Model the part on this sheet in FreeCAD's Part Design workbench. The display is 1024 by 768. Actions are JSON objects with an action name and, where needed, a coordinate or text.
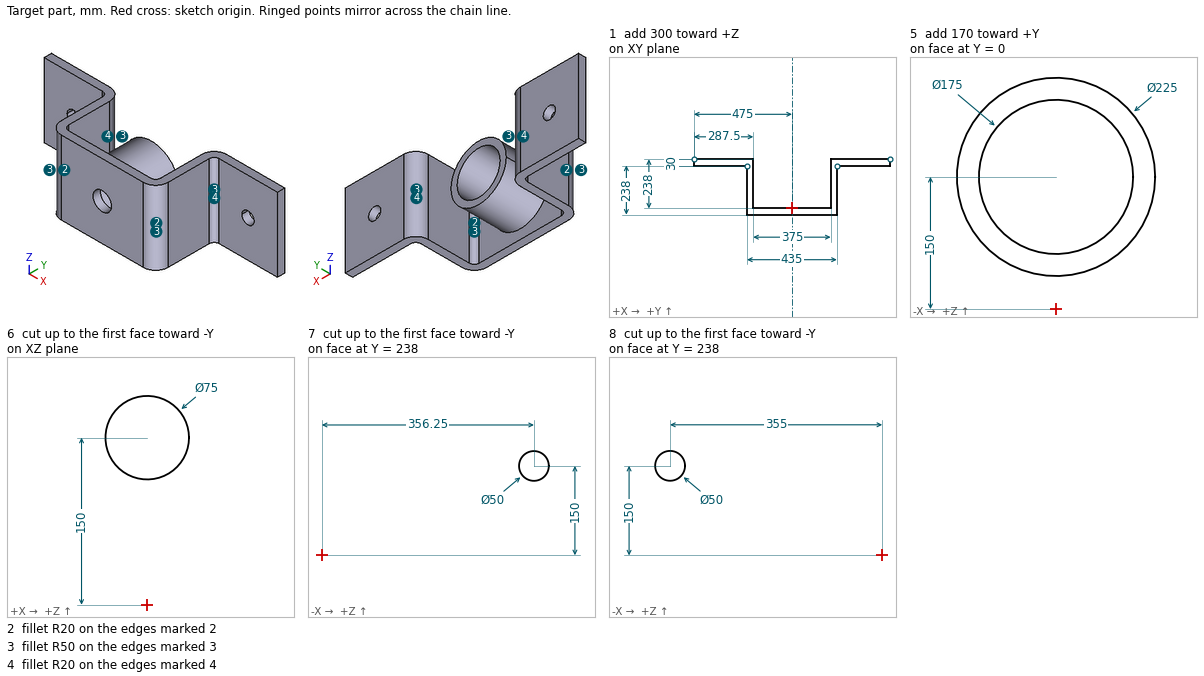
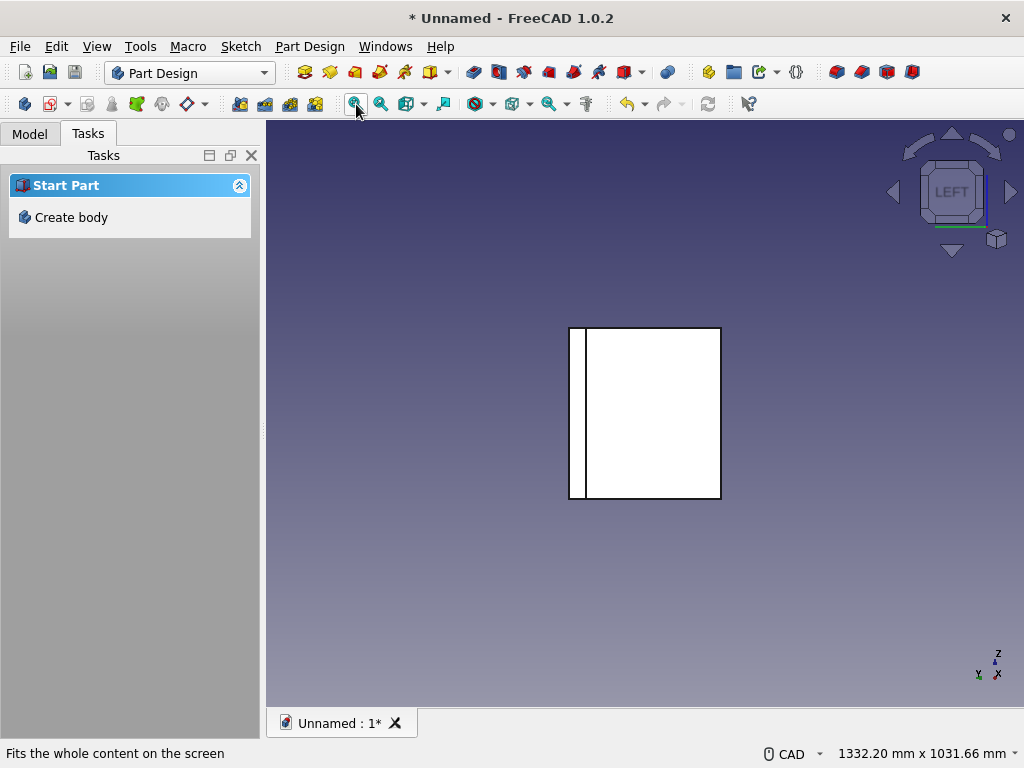
{"action": "key", "text": "v 3"}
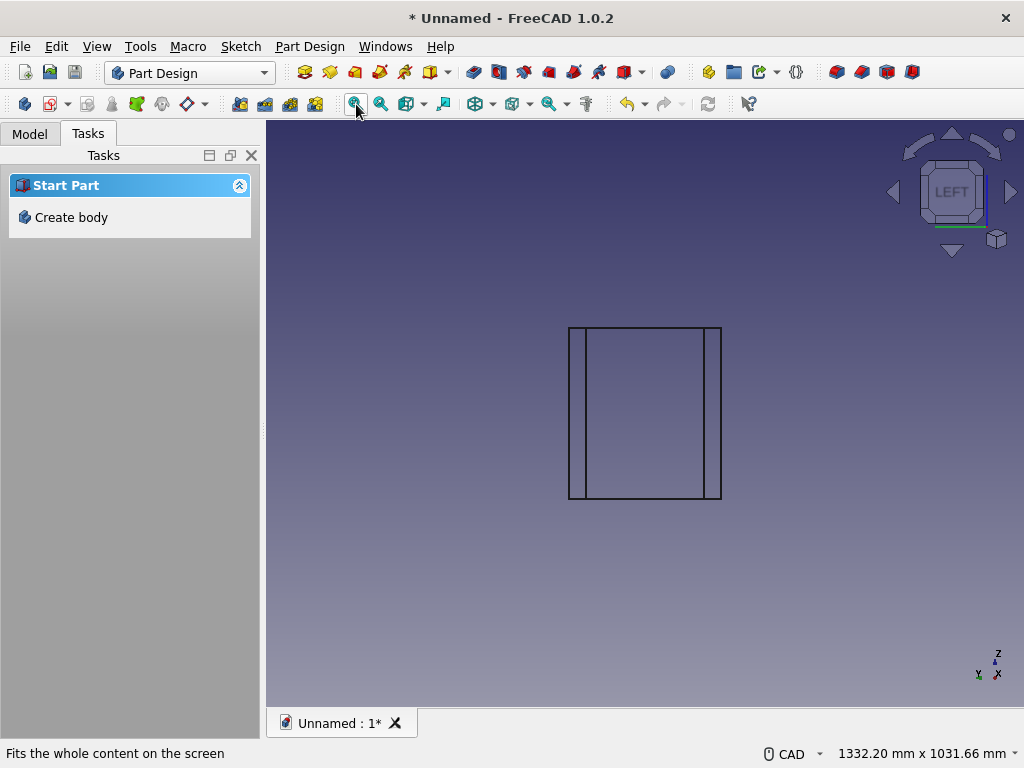
{"action": "key", "text": "0"}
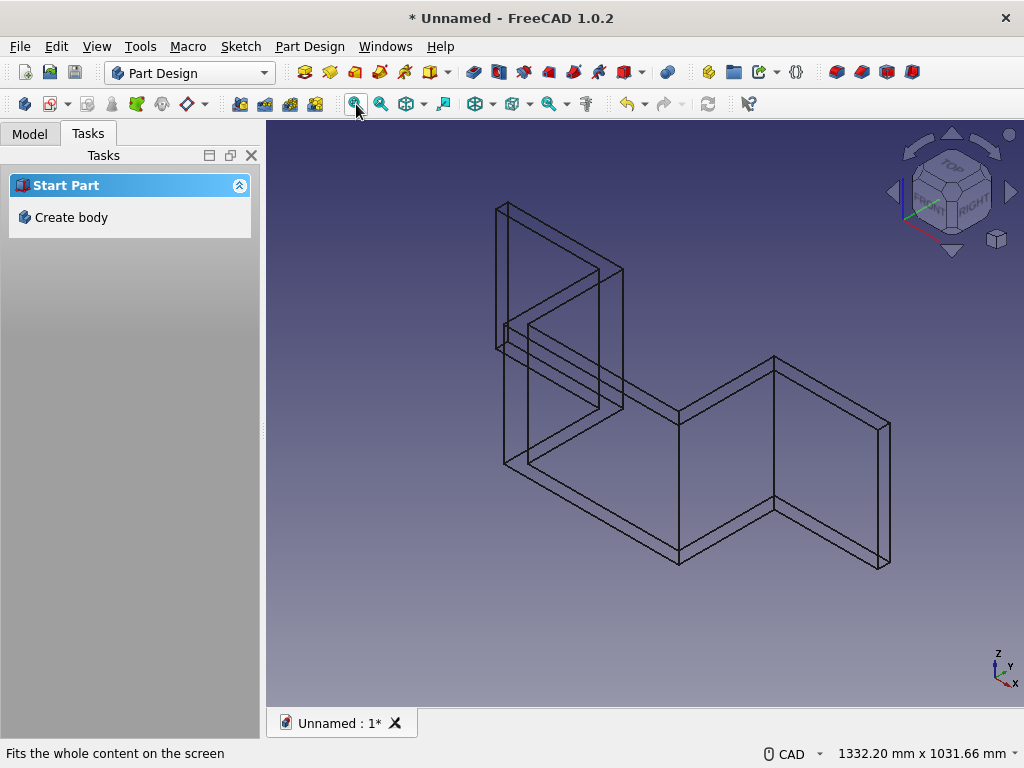
{"action": "left_click", "coordinate": [528, 393]}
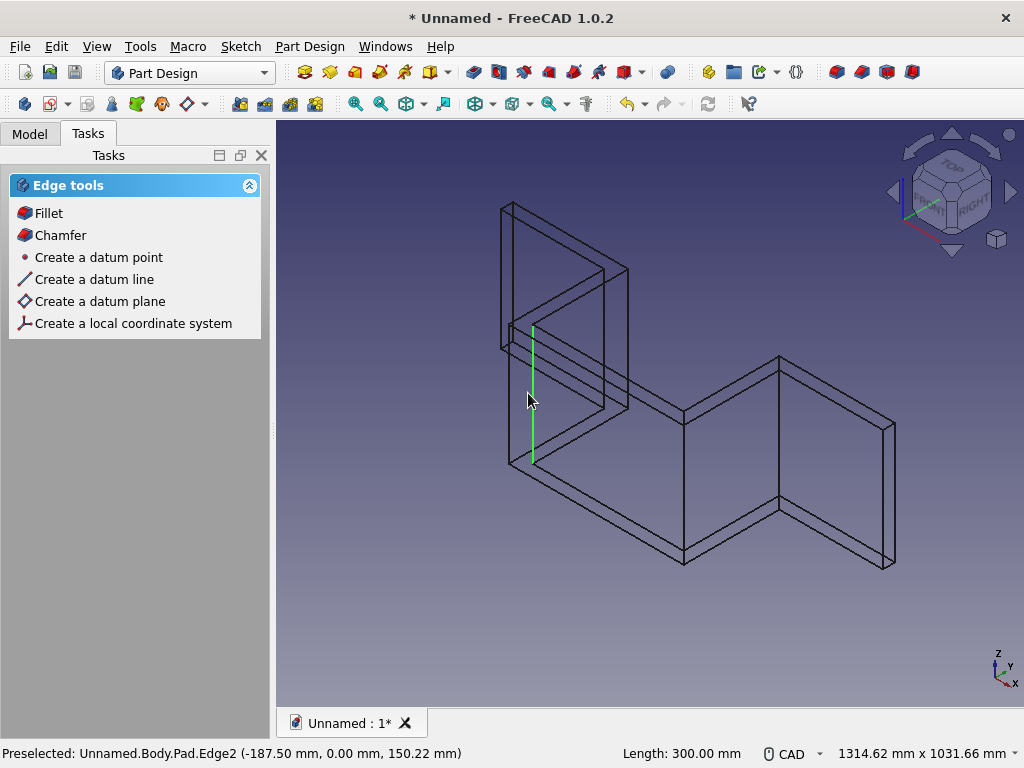
{"action": "scroll", "coordinate": [684, 480], "scroll_direction": "up", "scroll_amount": 6}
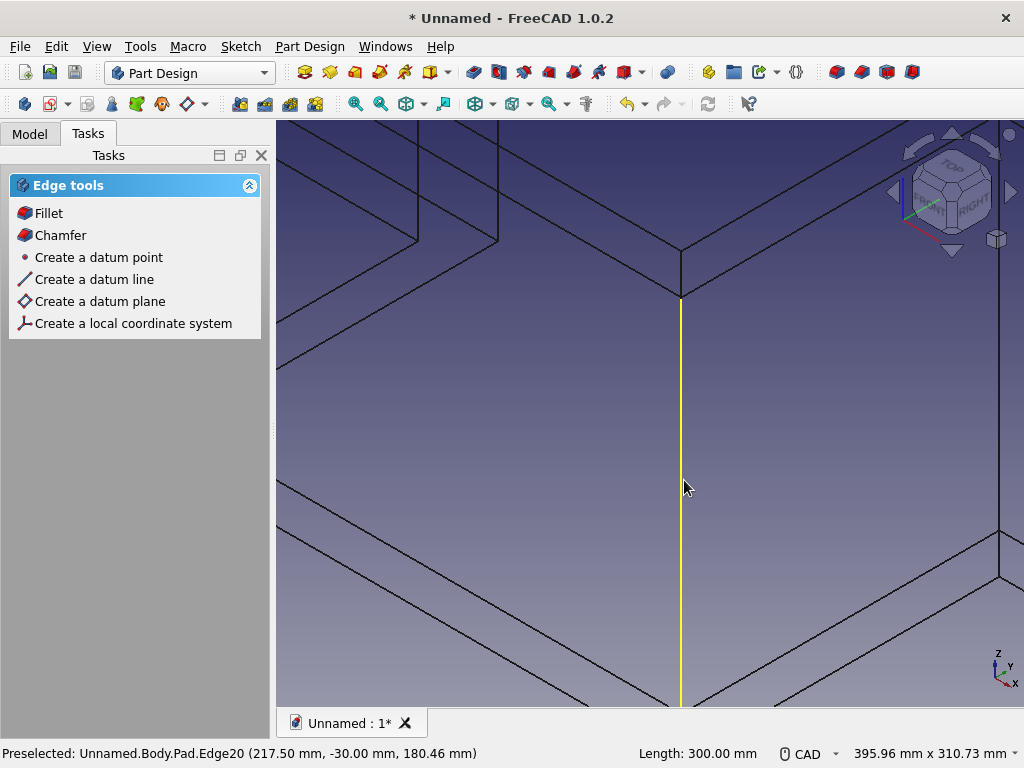
{"action": "left_click", "coordinate": [356, 104]}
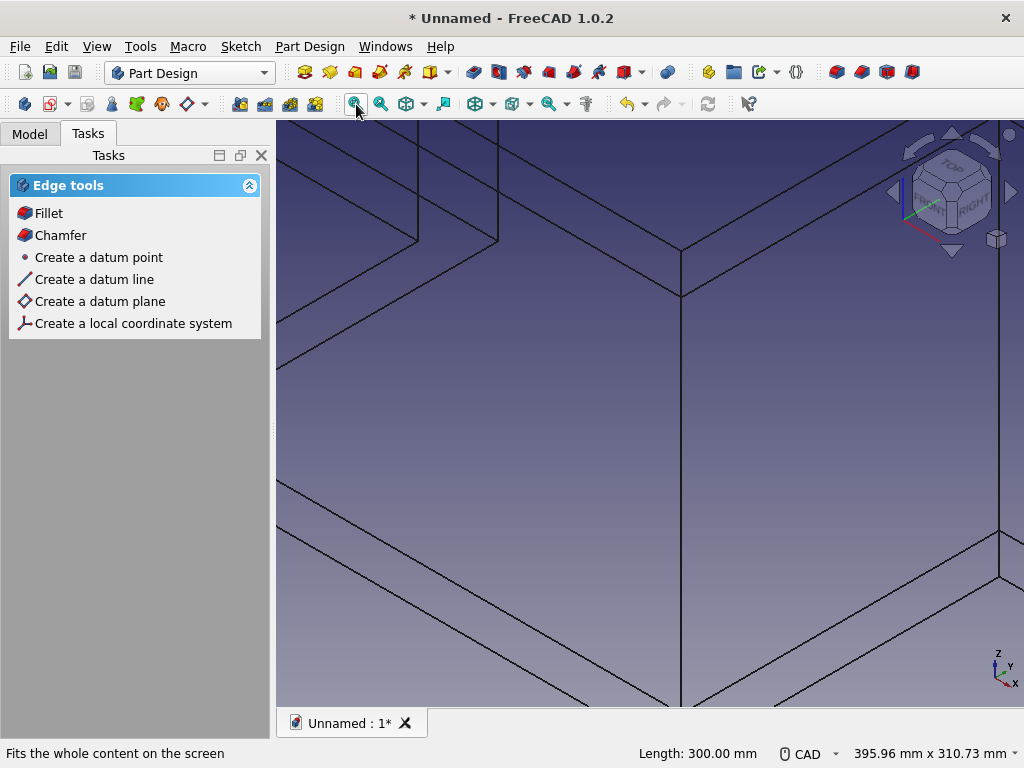
{"action": "key", "text": "2"}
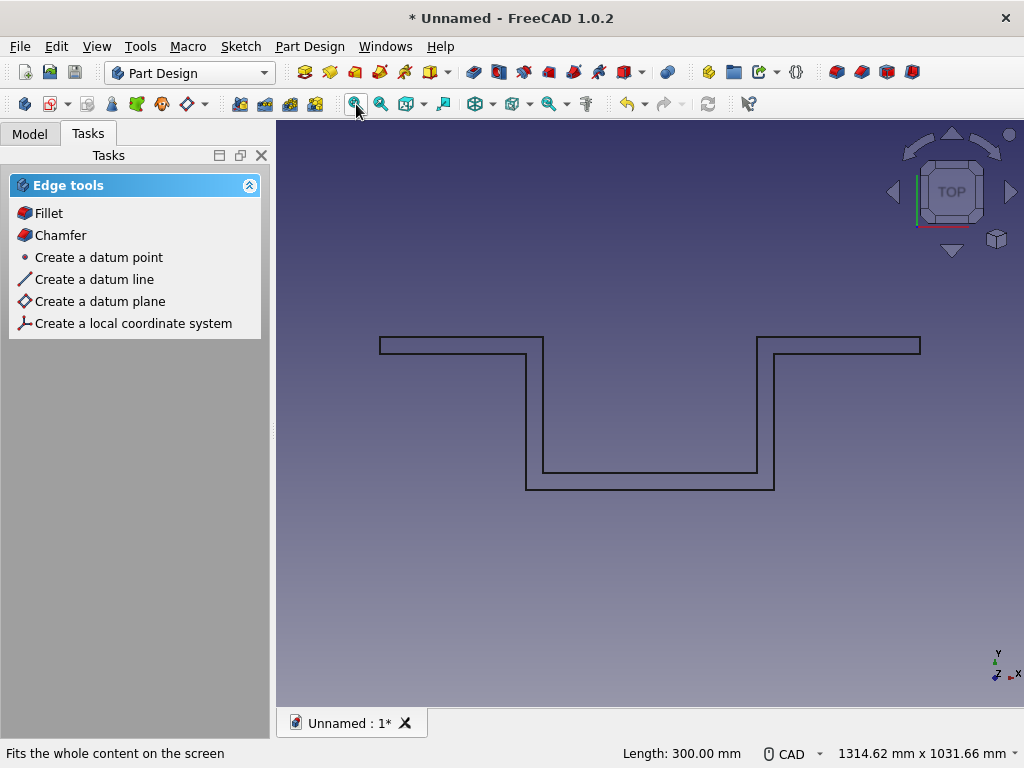
{"action": "scroll", "coordinate": [757, 472], "scroll_direction": "up", "scroll_amount": 6}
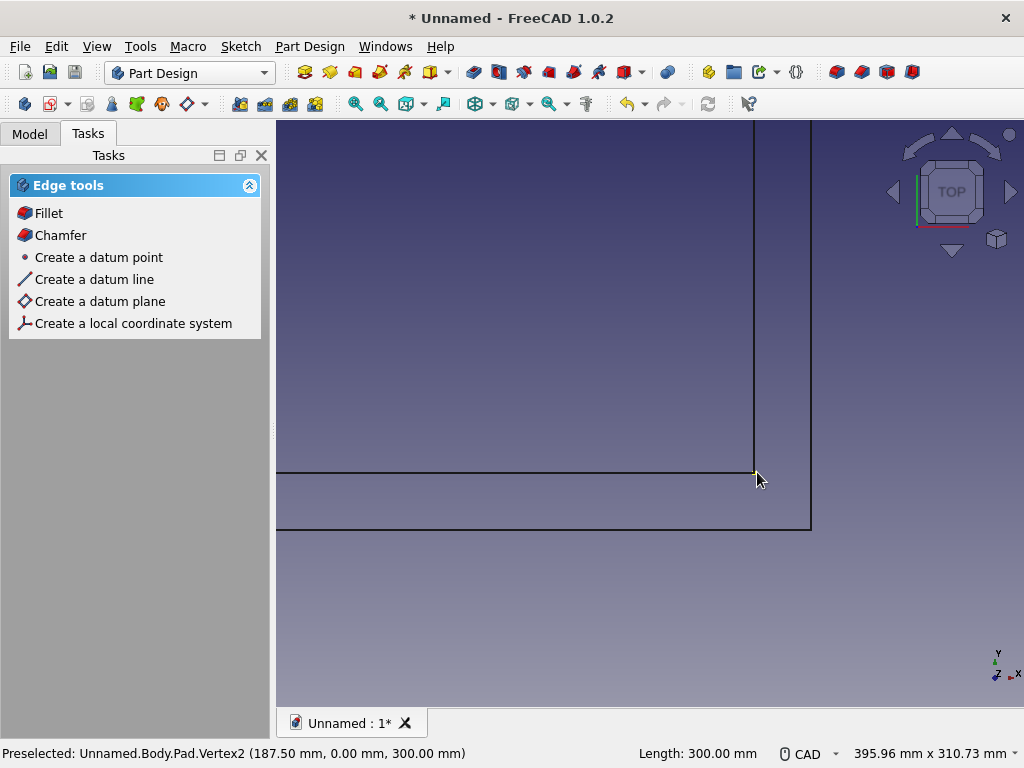
{"action": "left_click", "coordinate": [356, 104]}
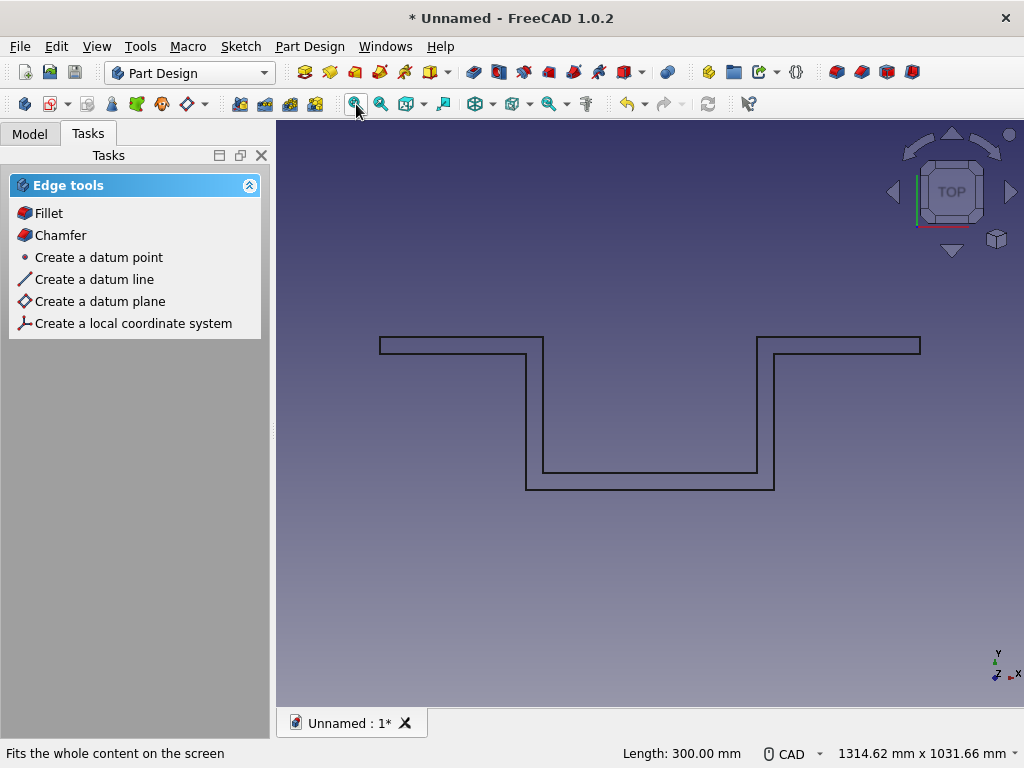
{"action": "key", "text": "1"}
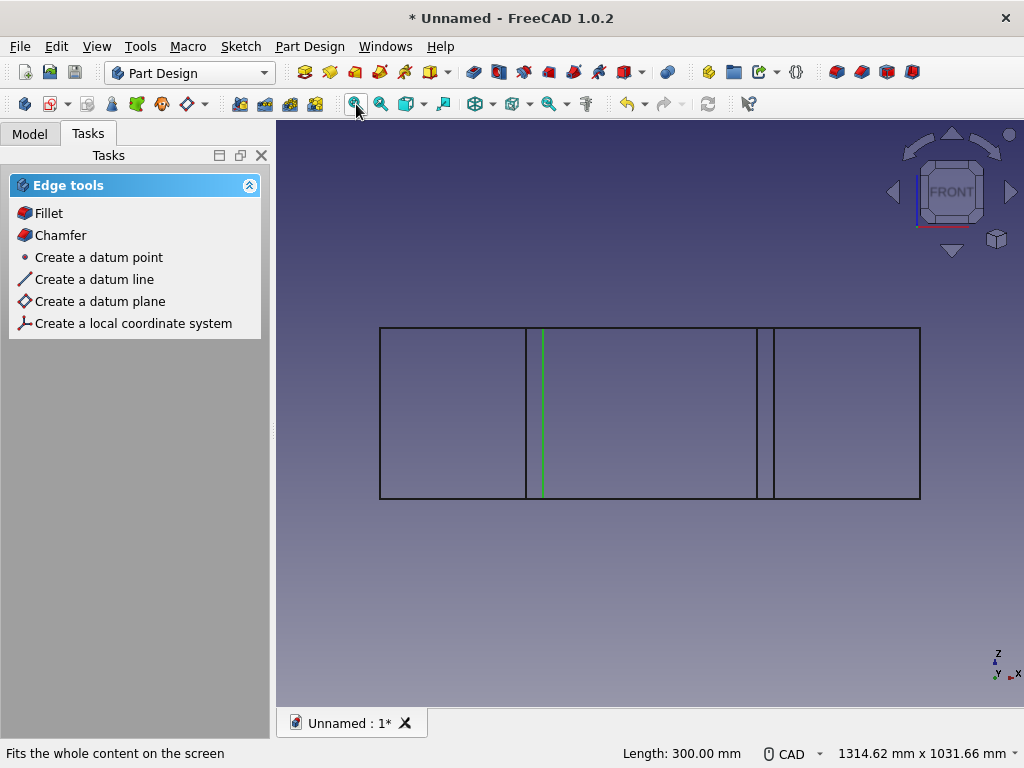
{"action": "left_click", "coordinate": [757, 412], "text": "ctrl"}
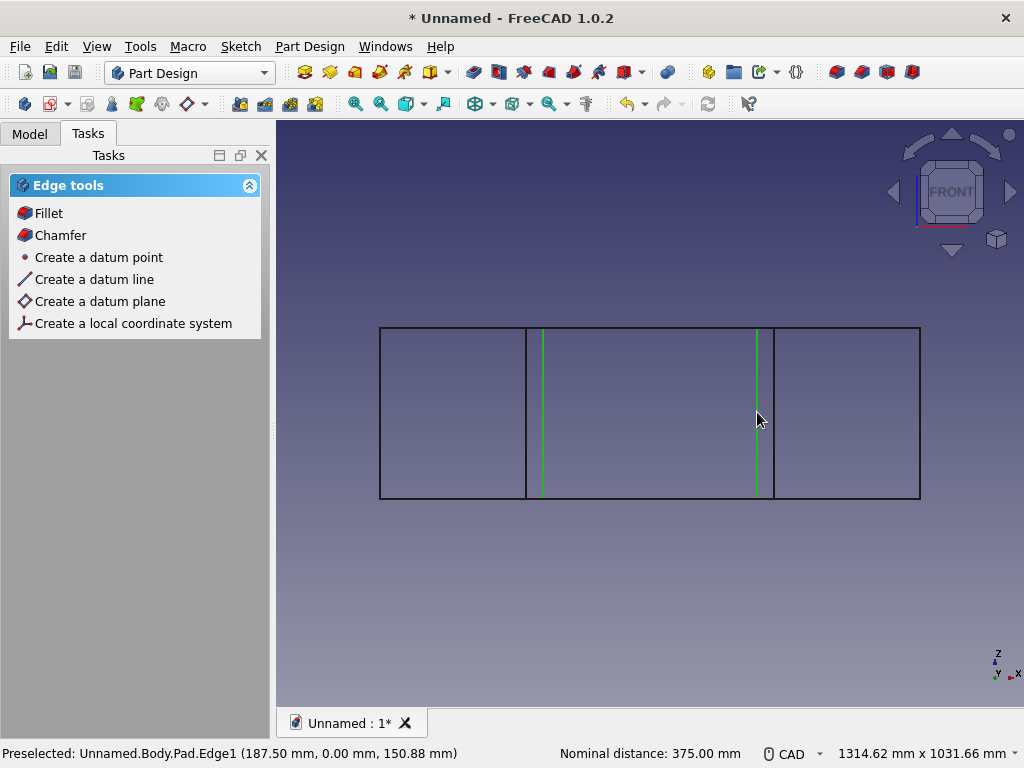
{"action": "key", "text": "v 1"}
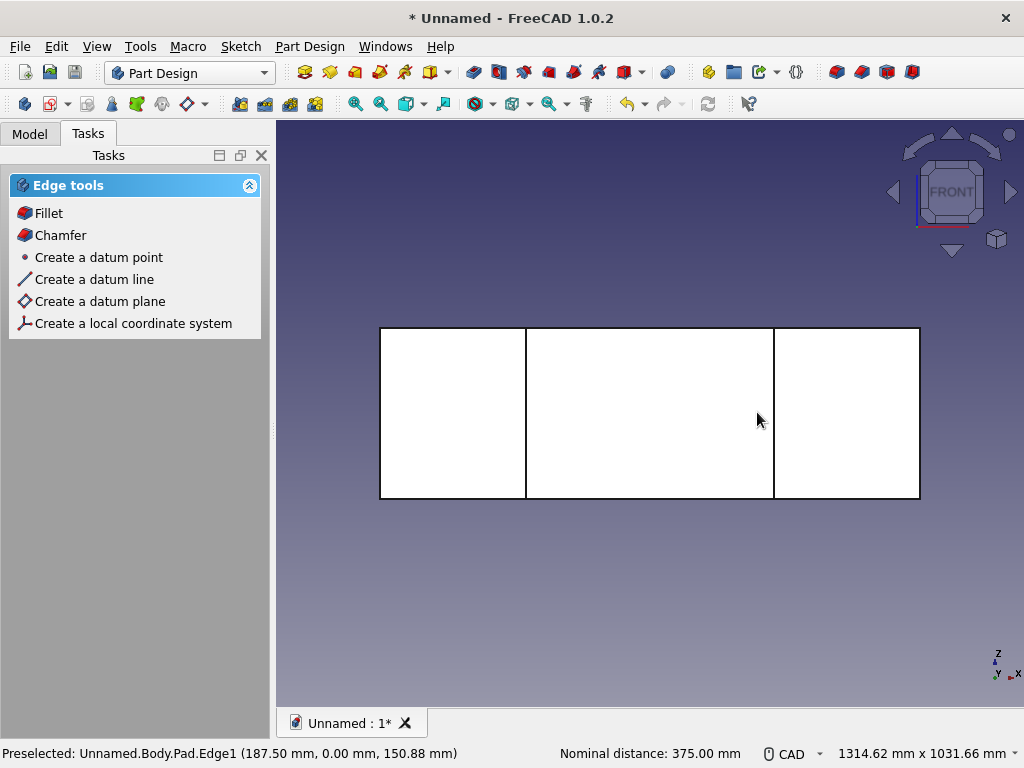
{"action": "left_click", "coordinate": [837, 72]}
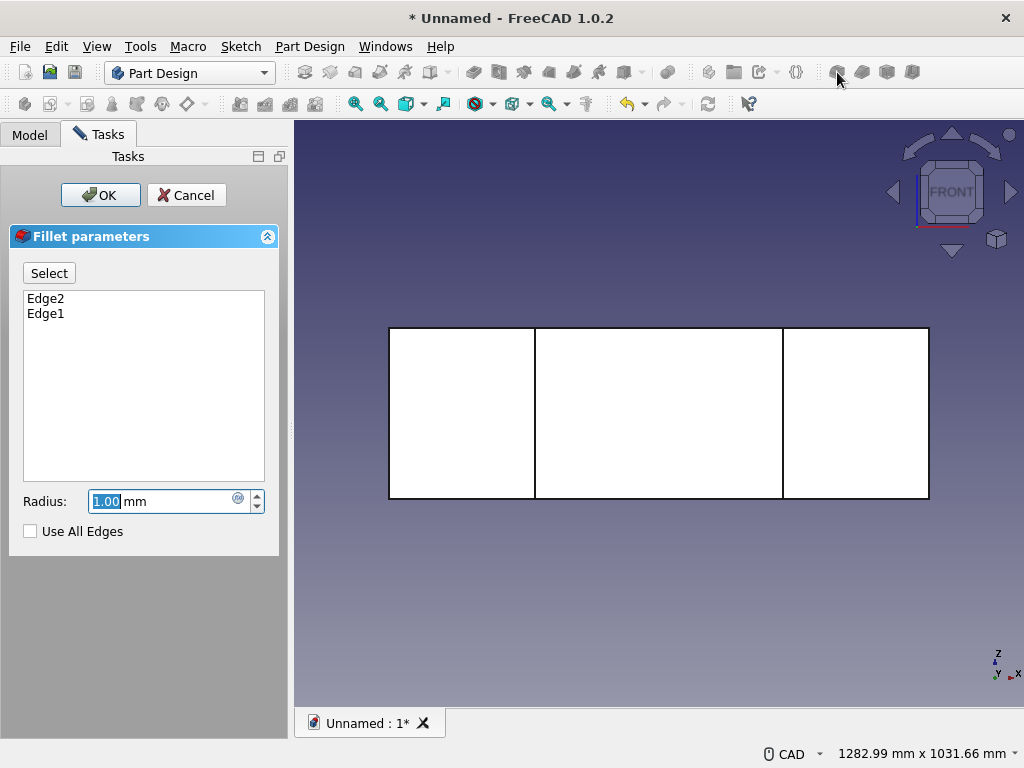
{"action": "type", "text": "20"}
{"action": "key", "text": "Tab"}